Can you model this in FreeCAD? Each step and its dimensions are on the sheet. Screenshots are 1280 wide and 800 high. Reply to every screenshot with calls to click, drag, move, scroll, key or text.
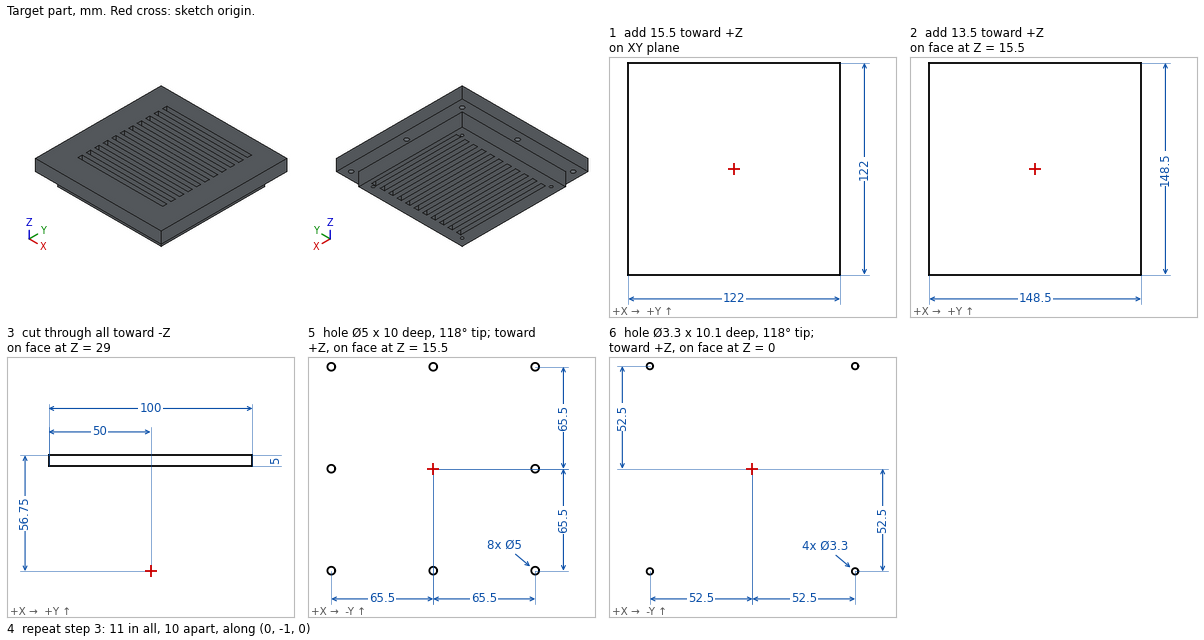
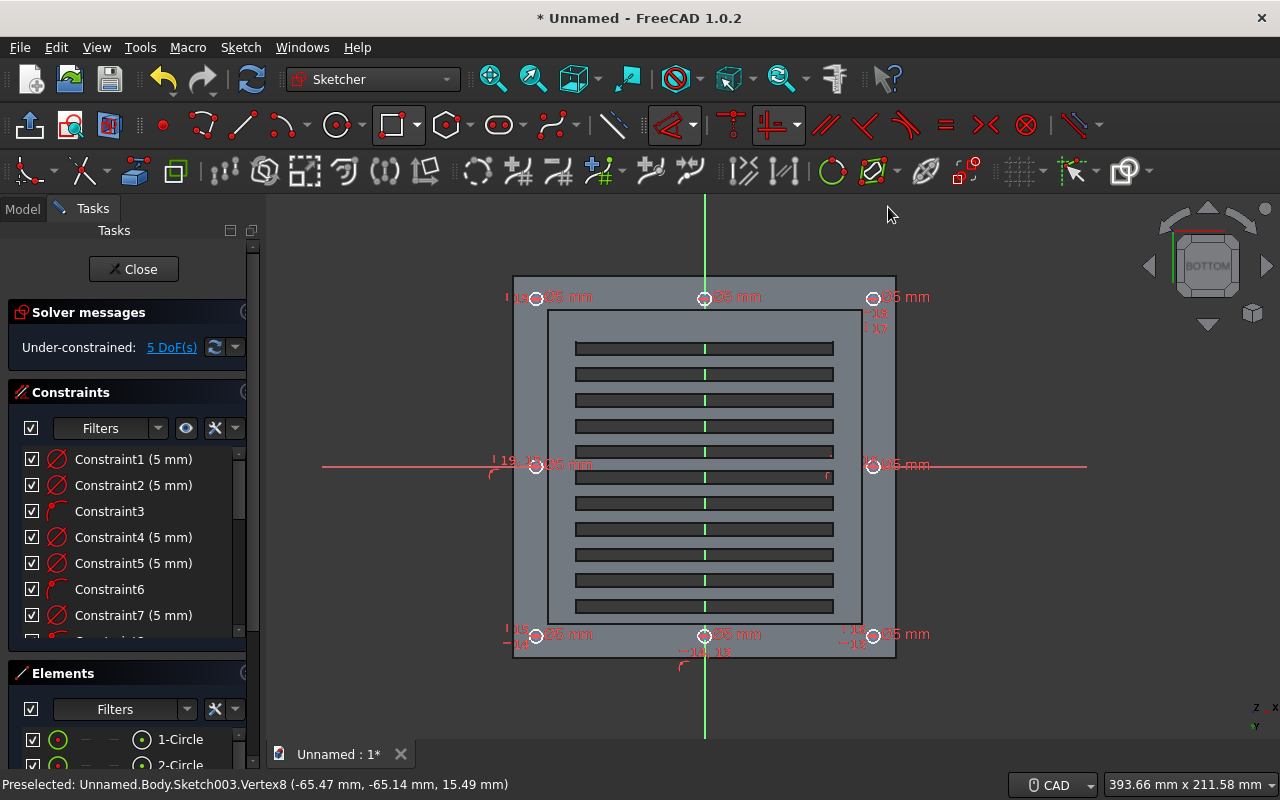
click(705, 299)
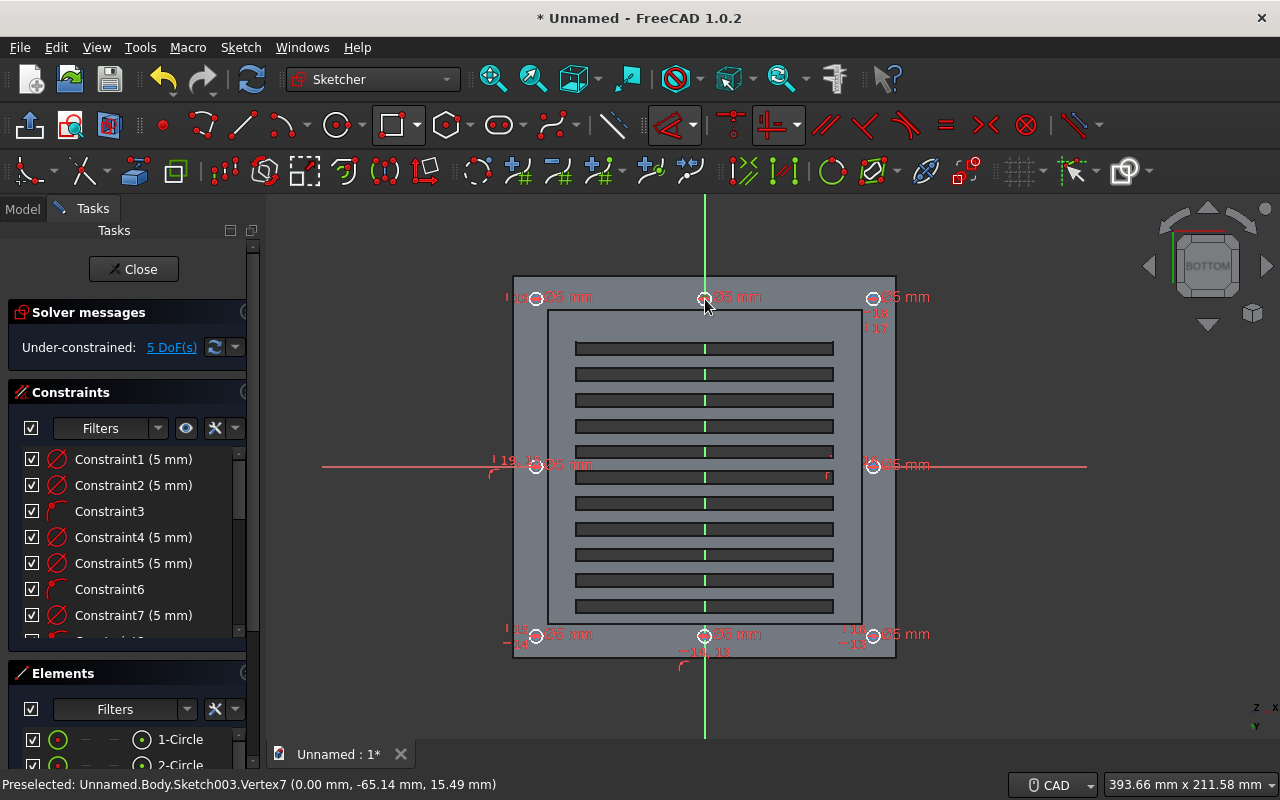
click(536, 299)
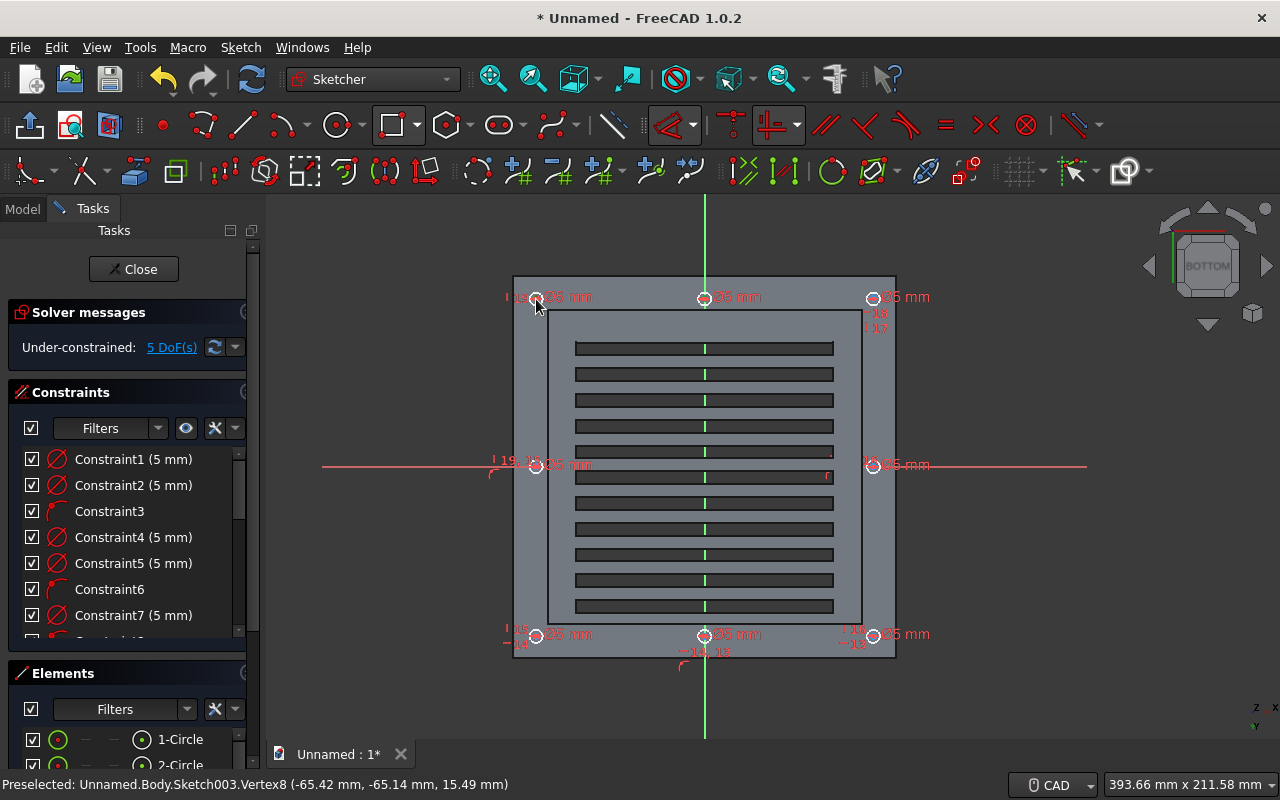
key(h)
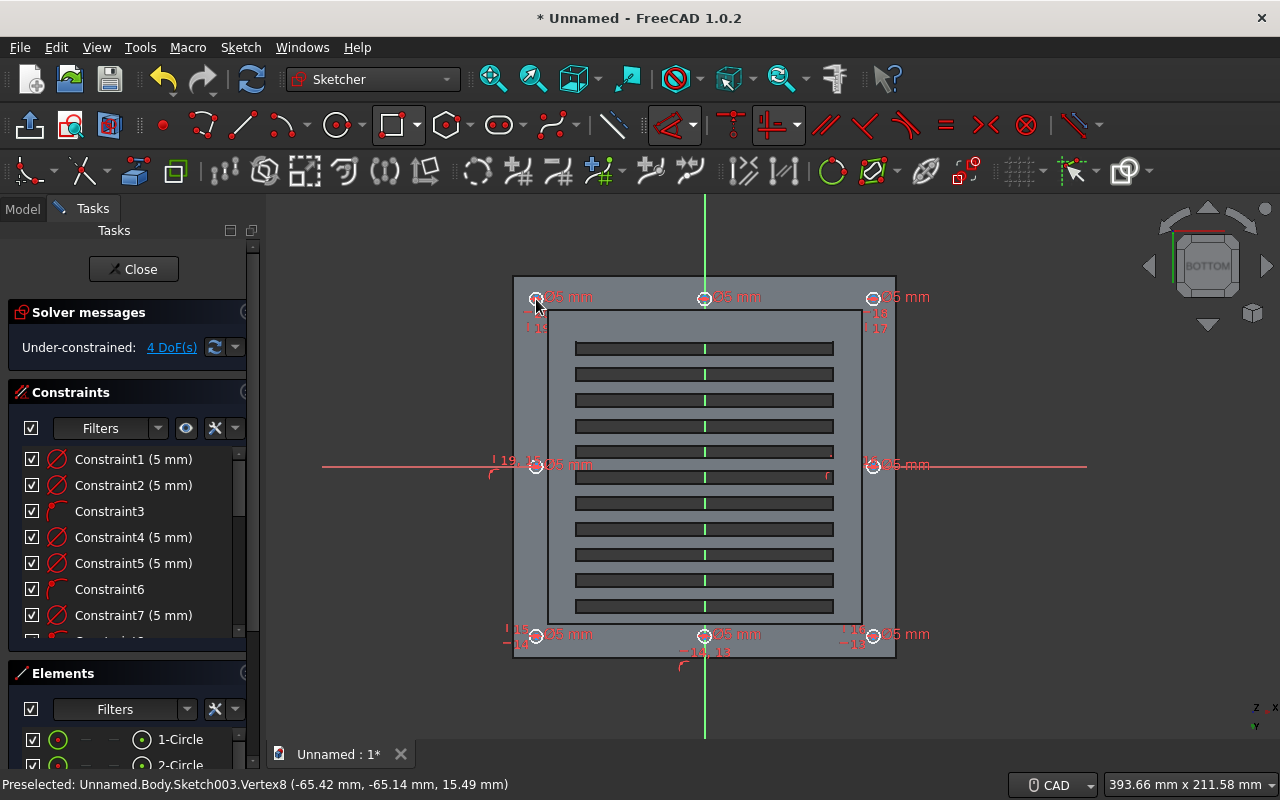
click(873, 636)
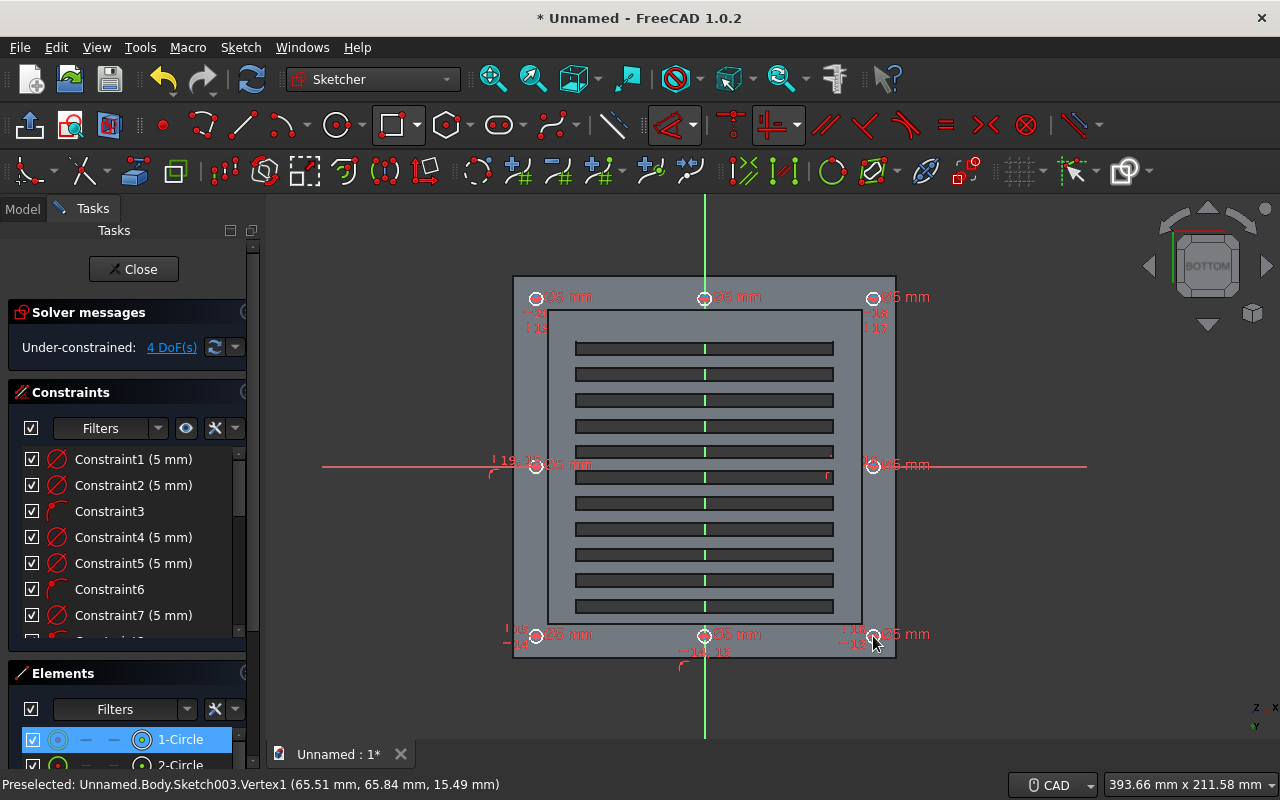
key(l)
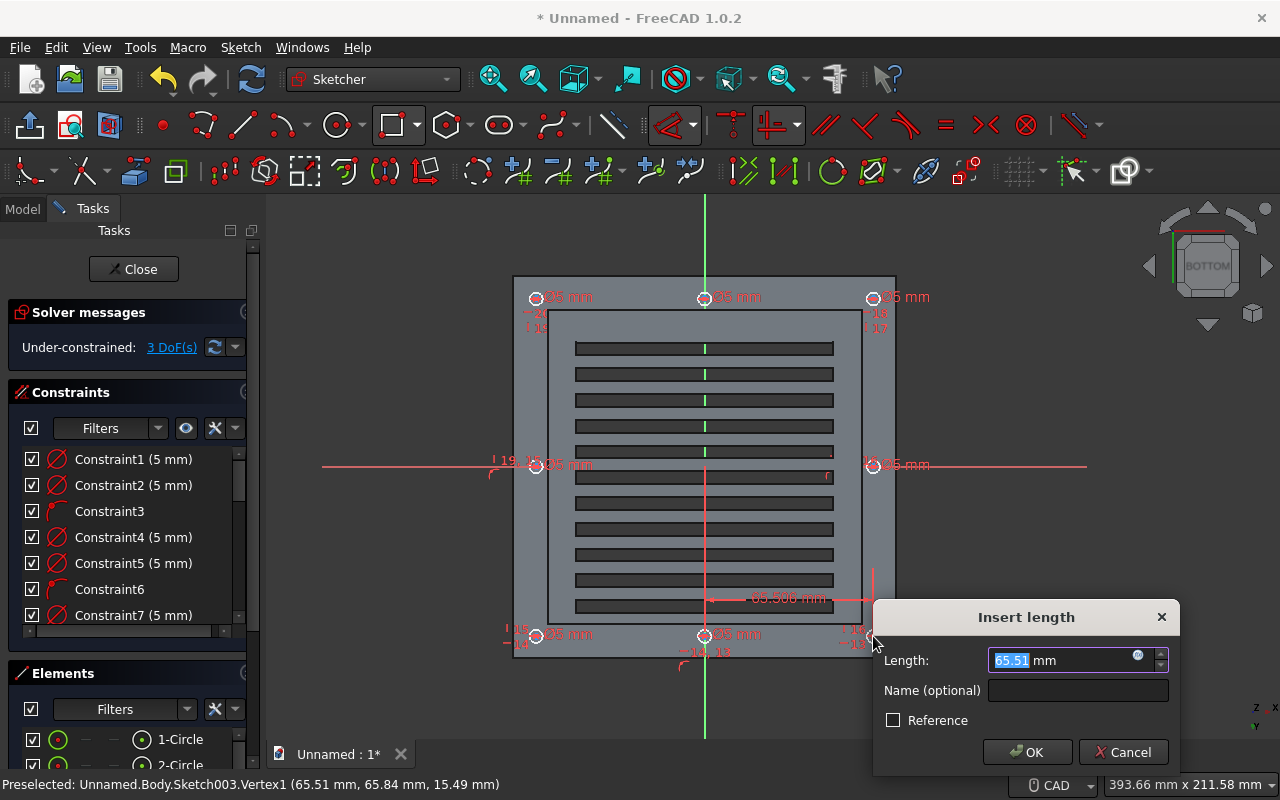
text(65.5)
key(Return)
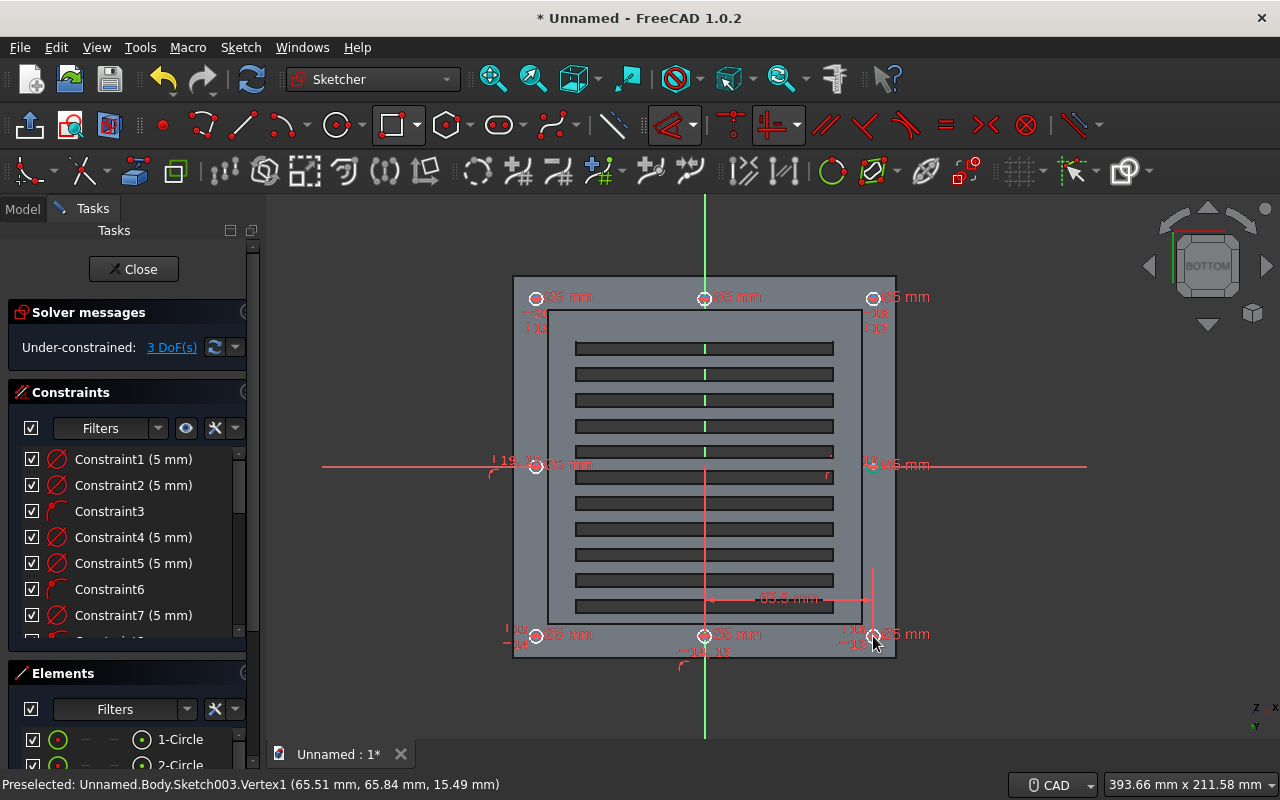
click(873, 636)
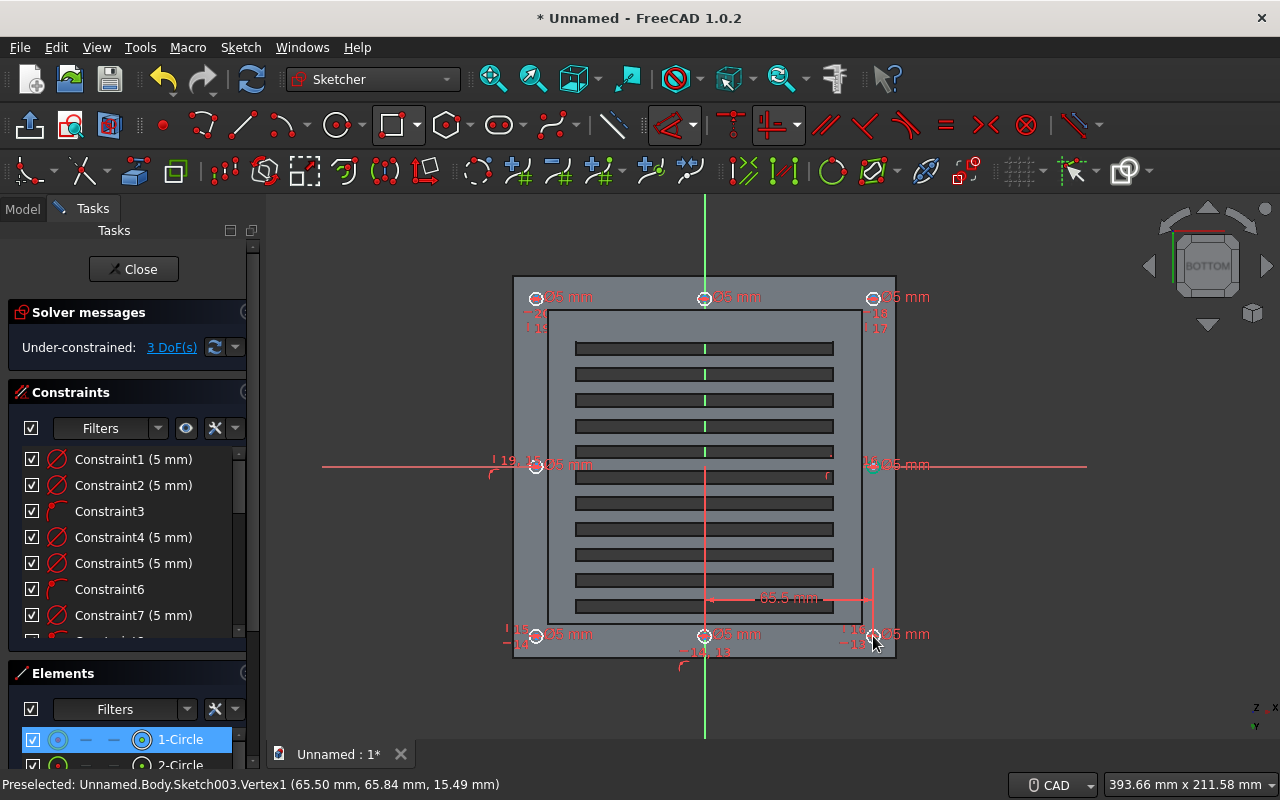
key(i)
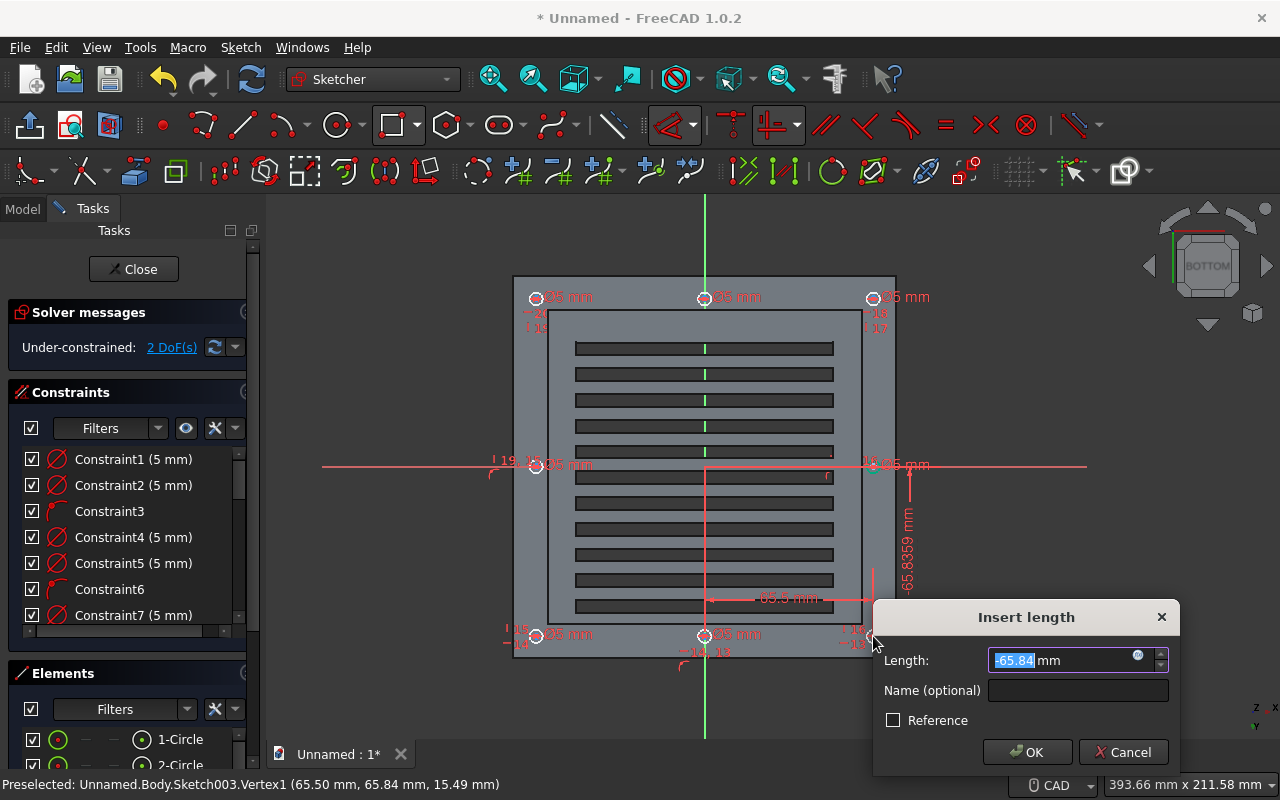
text(-65.5)
key(Return)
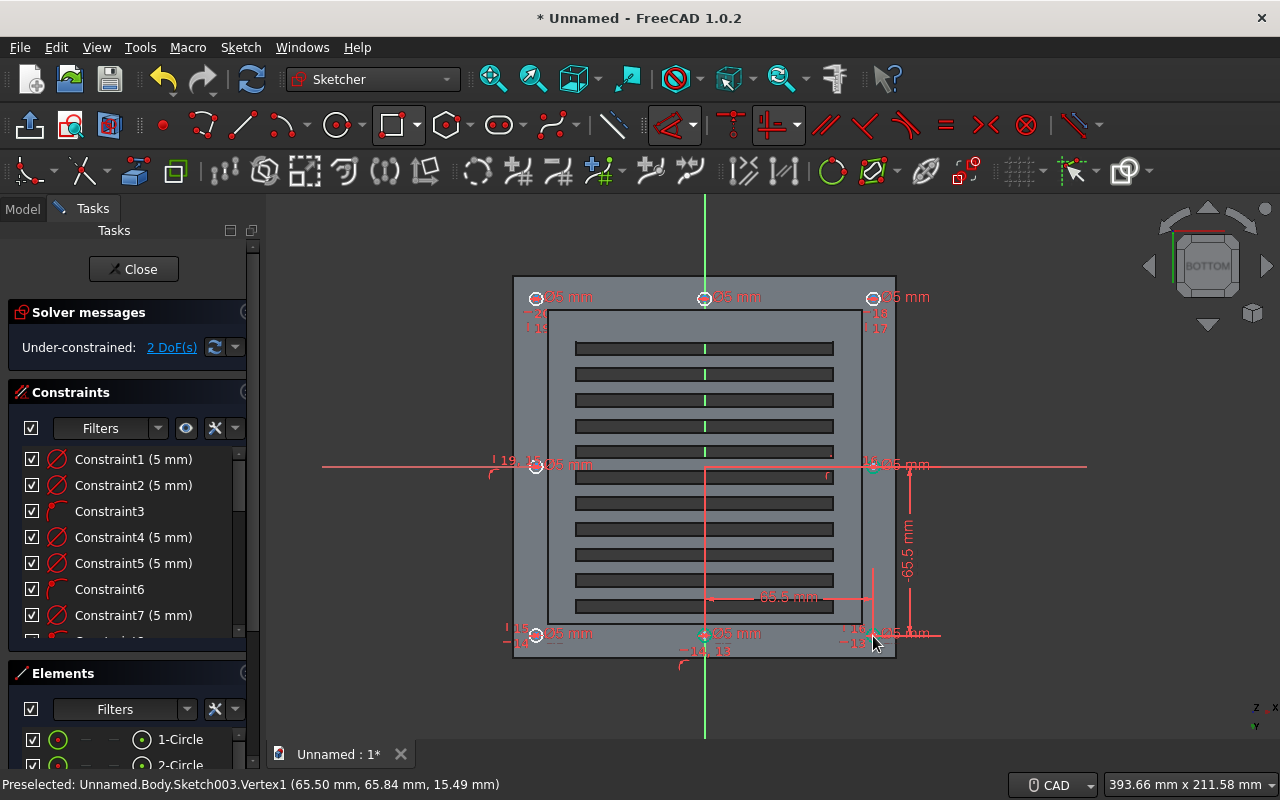
click(536, 636)